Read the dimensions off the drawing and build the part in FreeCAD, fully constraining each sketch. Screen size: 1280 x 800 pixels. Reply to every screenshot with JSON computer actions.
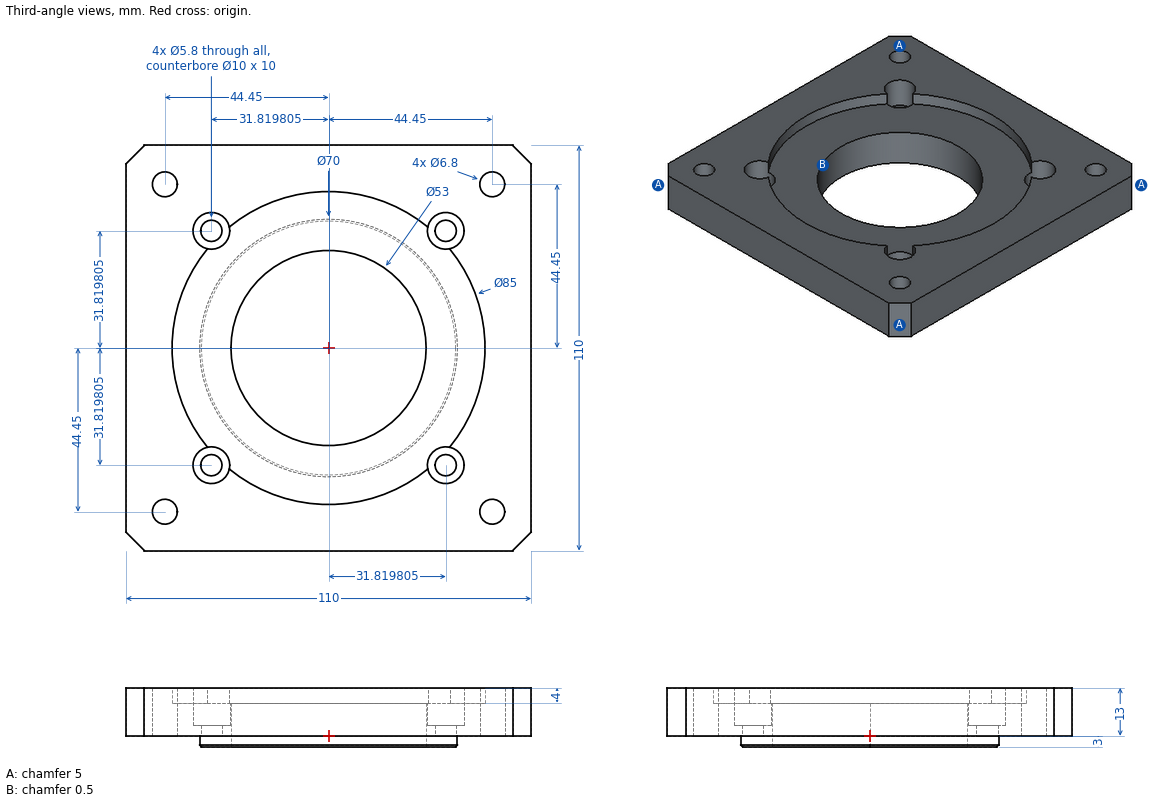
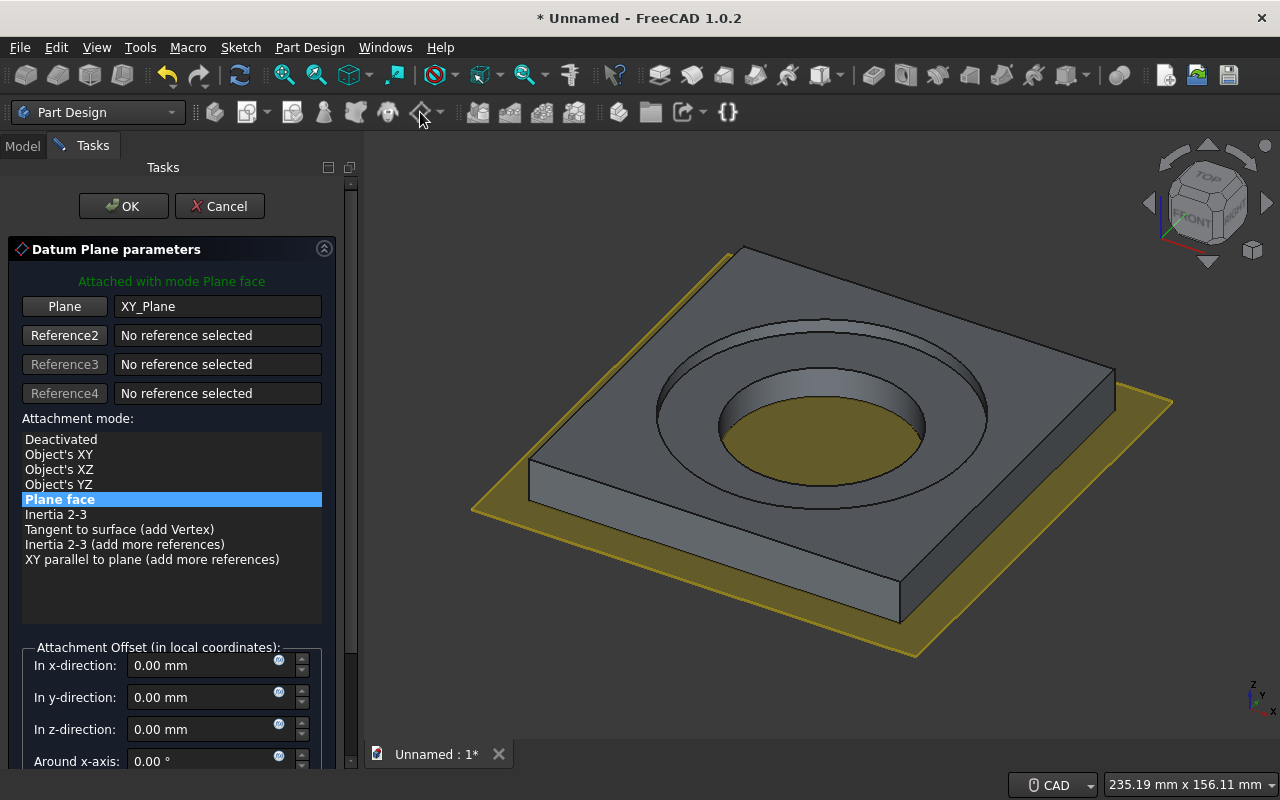
{"action": "triple_click", "coordinate": [210, 729]}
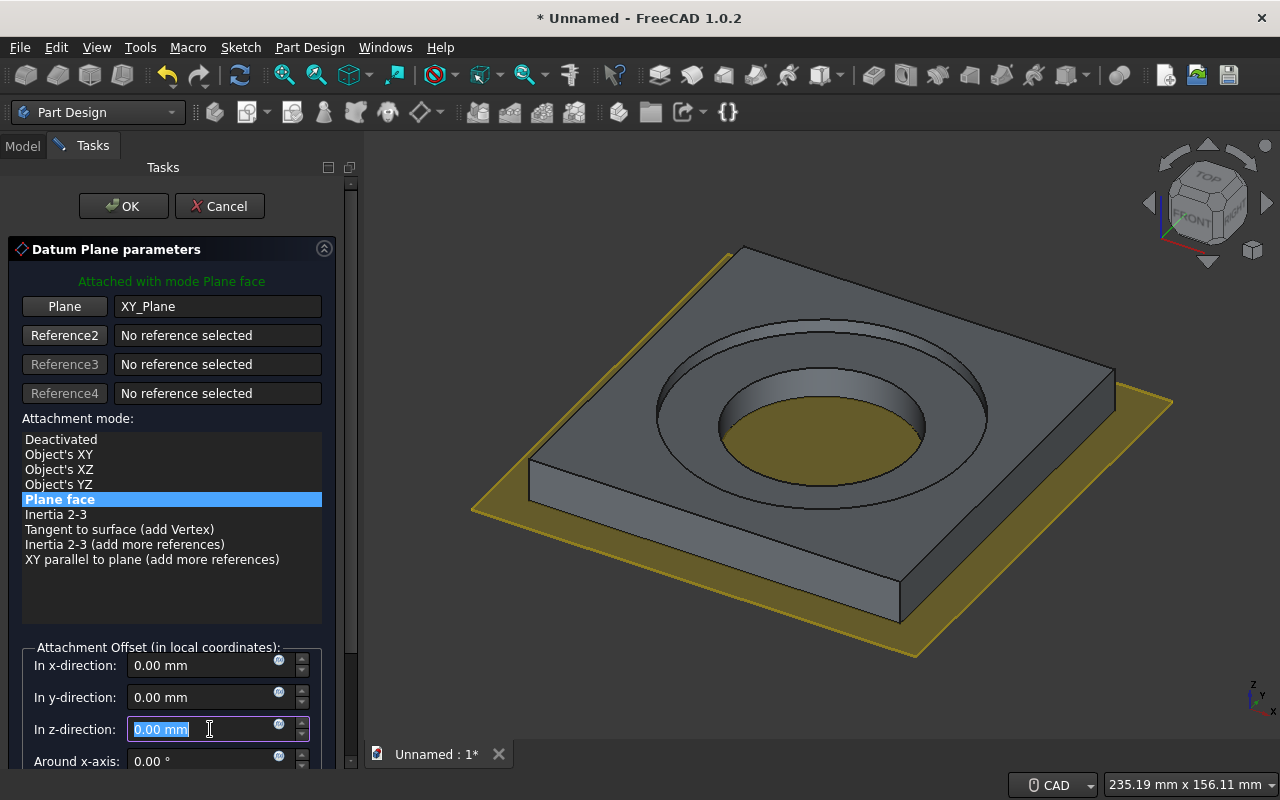
{"action": "type", "text": "-3"}
{"action": "key", "text": "Tab"}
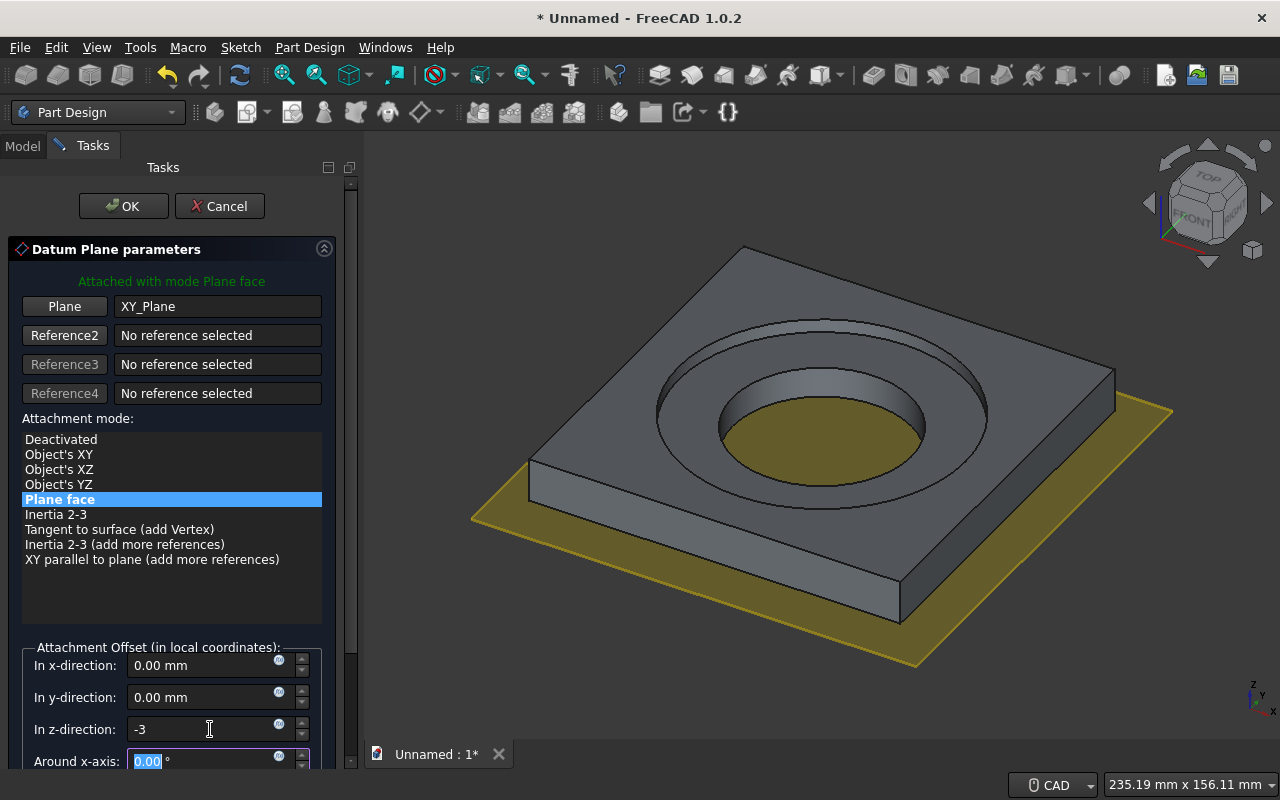
{"action": "left_click", "coordinate": [124, 206]}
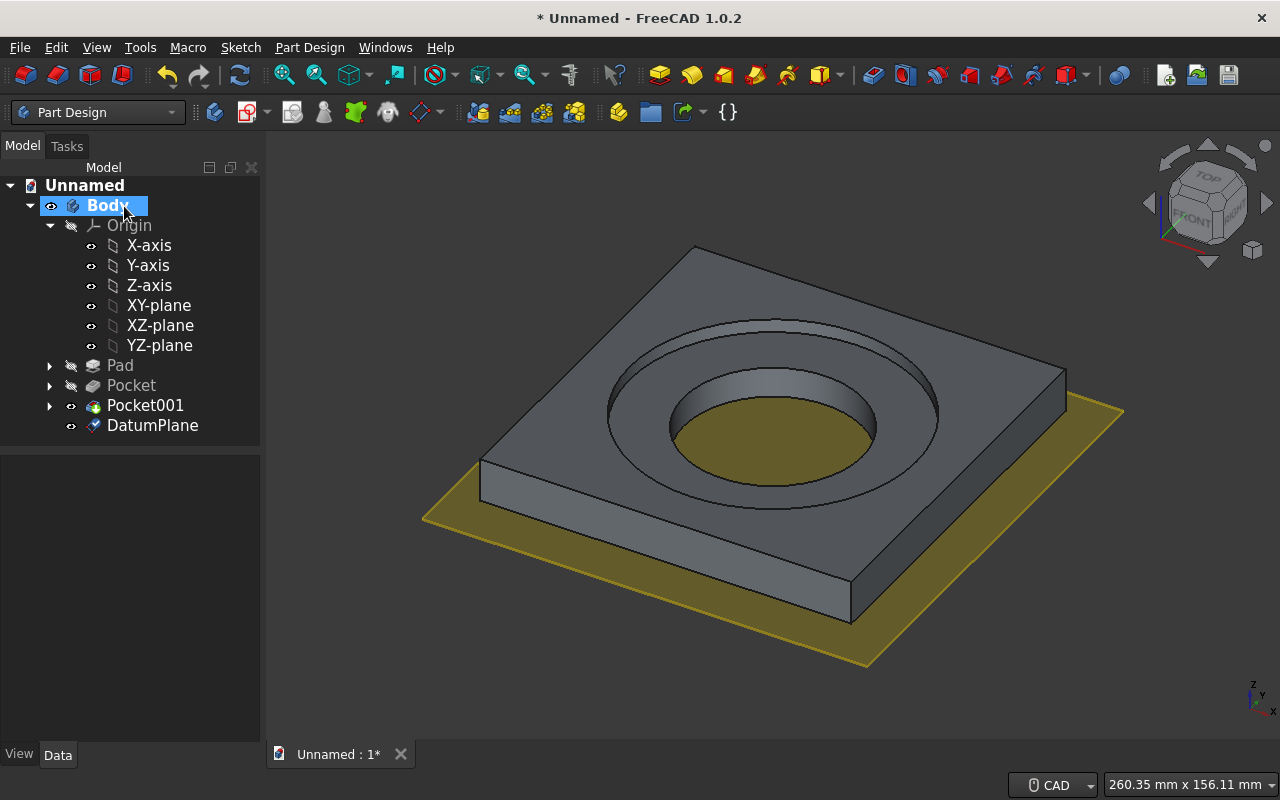
{"action": "left_click", "coordinate": [116, 426]}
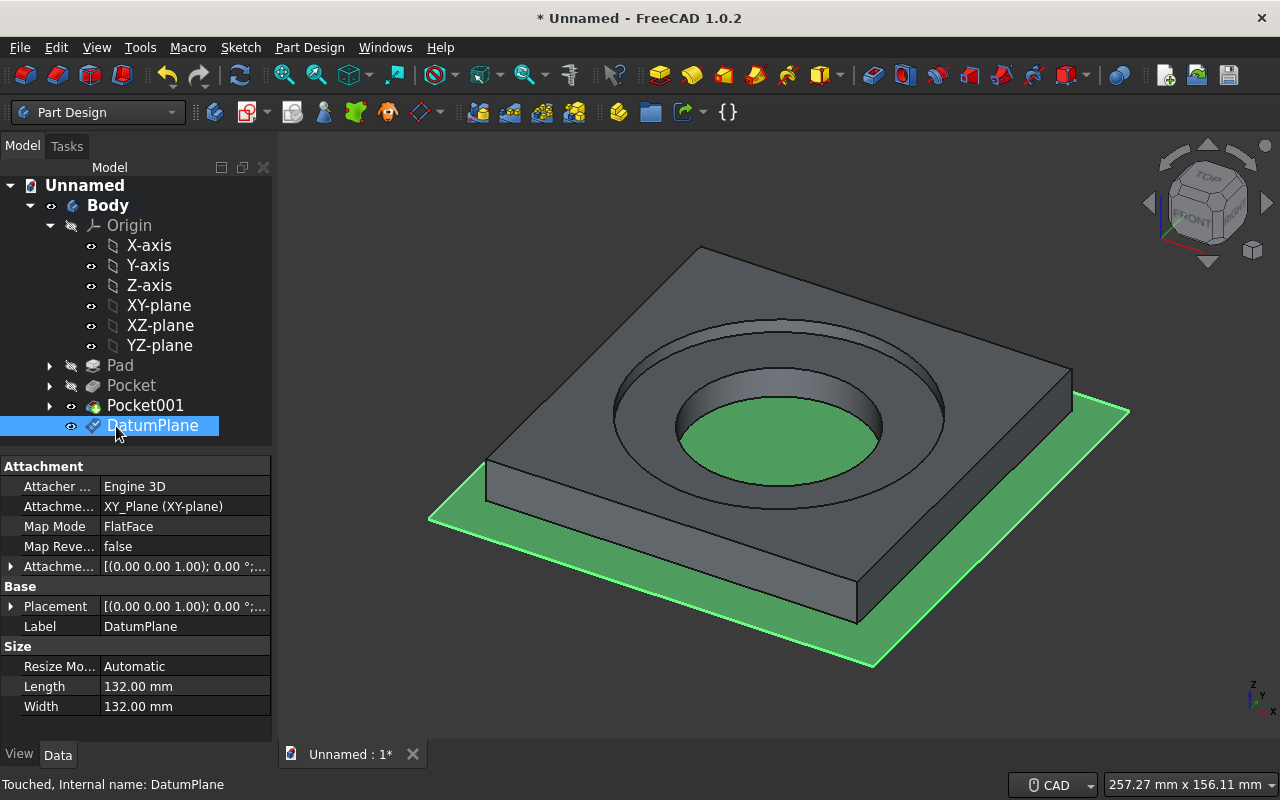
{"action": "left_click", "coordinate": [248, 112]}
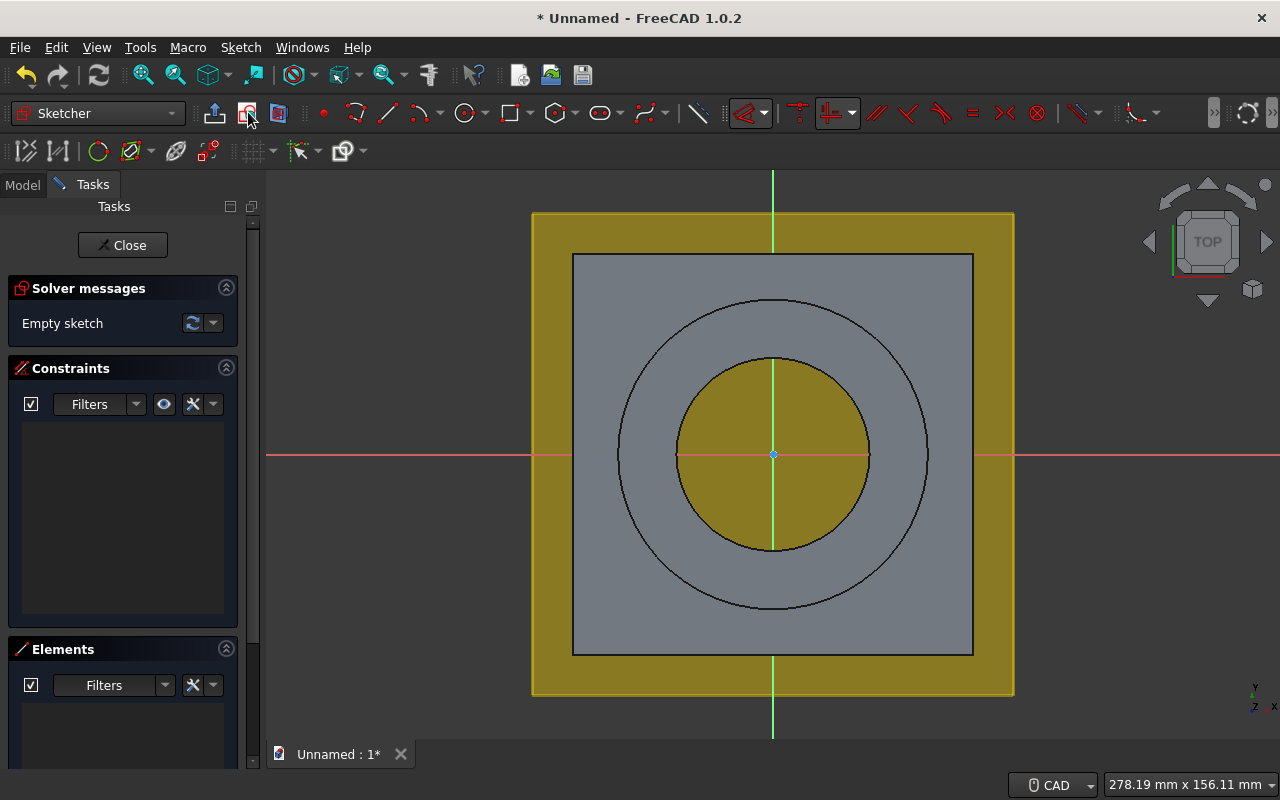
{"action": "left_click", "coordinate": [280, 114]}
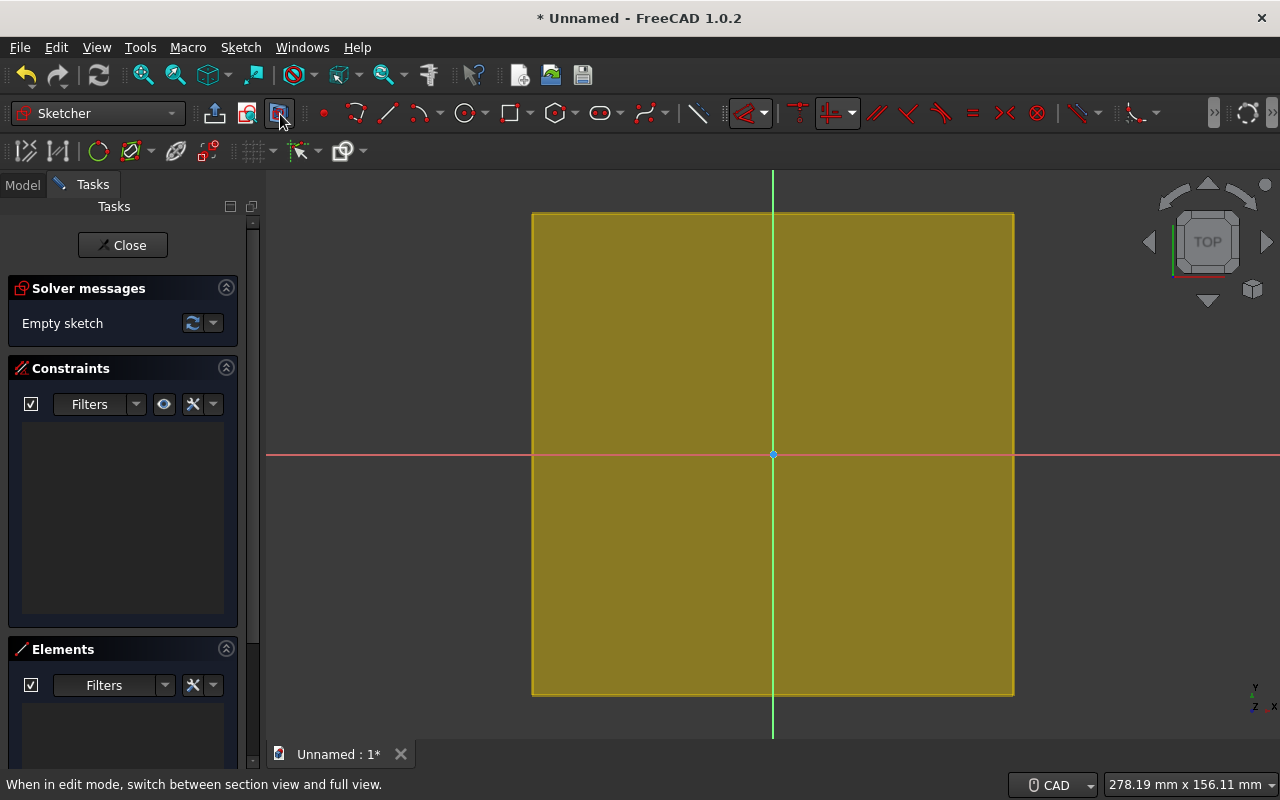
{"action": "scroll", "coordinate": [912, 455], "scroll_direction": "up", "scroll_amount": 2}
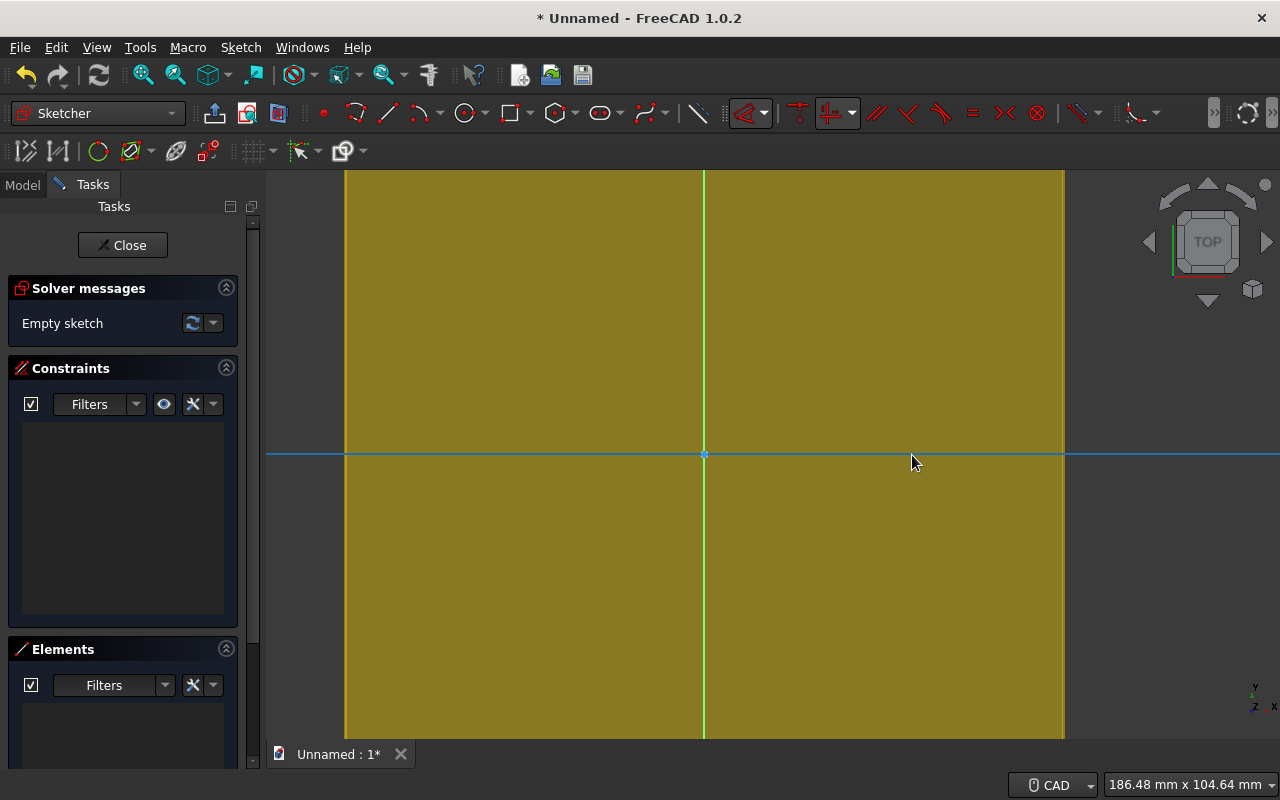
{"action": "key", "text": "g c"}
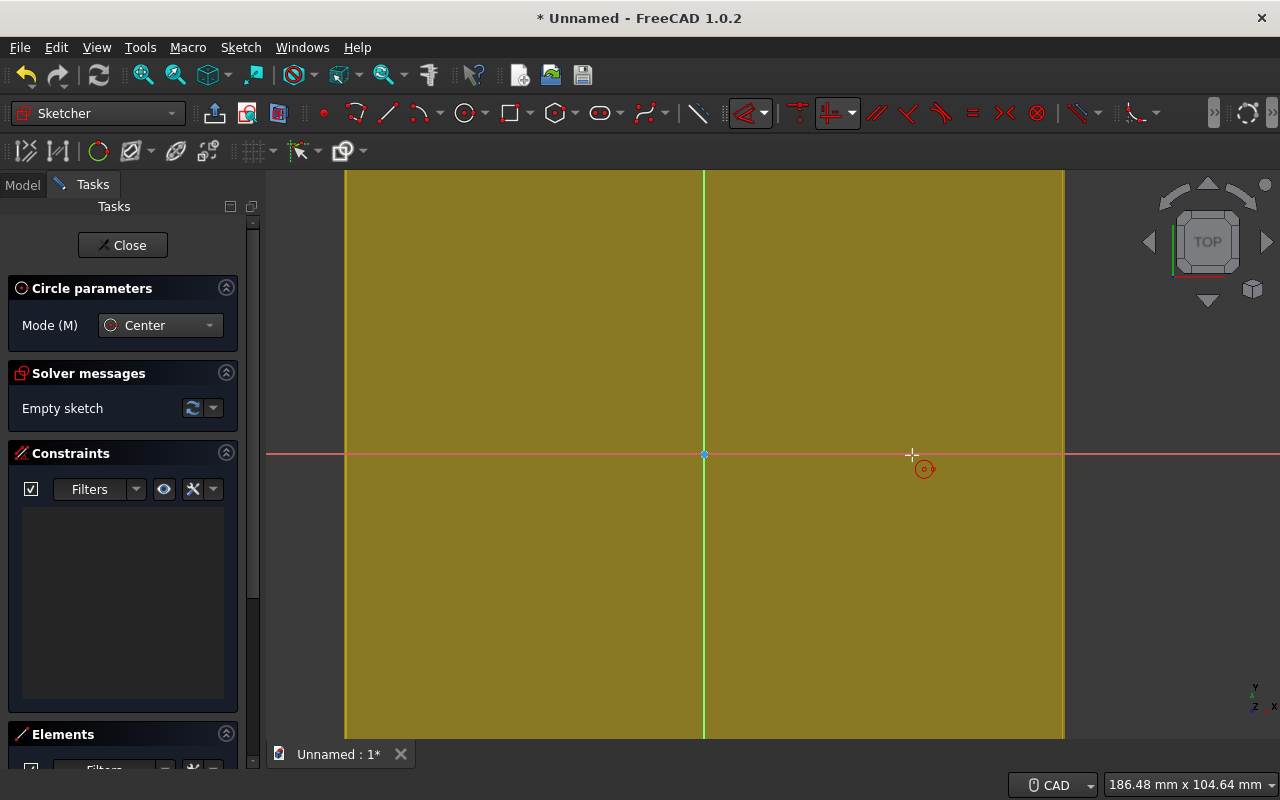
{"action": "left_click", "coordinate": [704, 454]}
{"action": "left_click", "coordinate": [839, 319]}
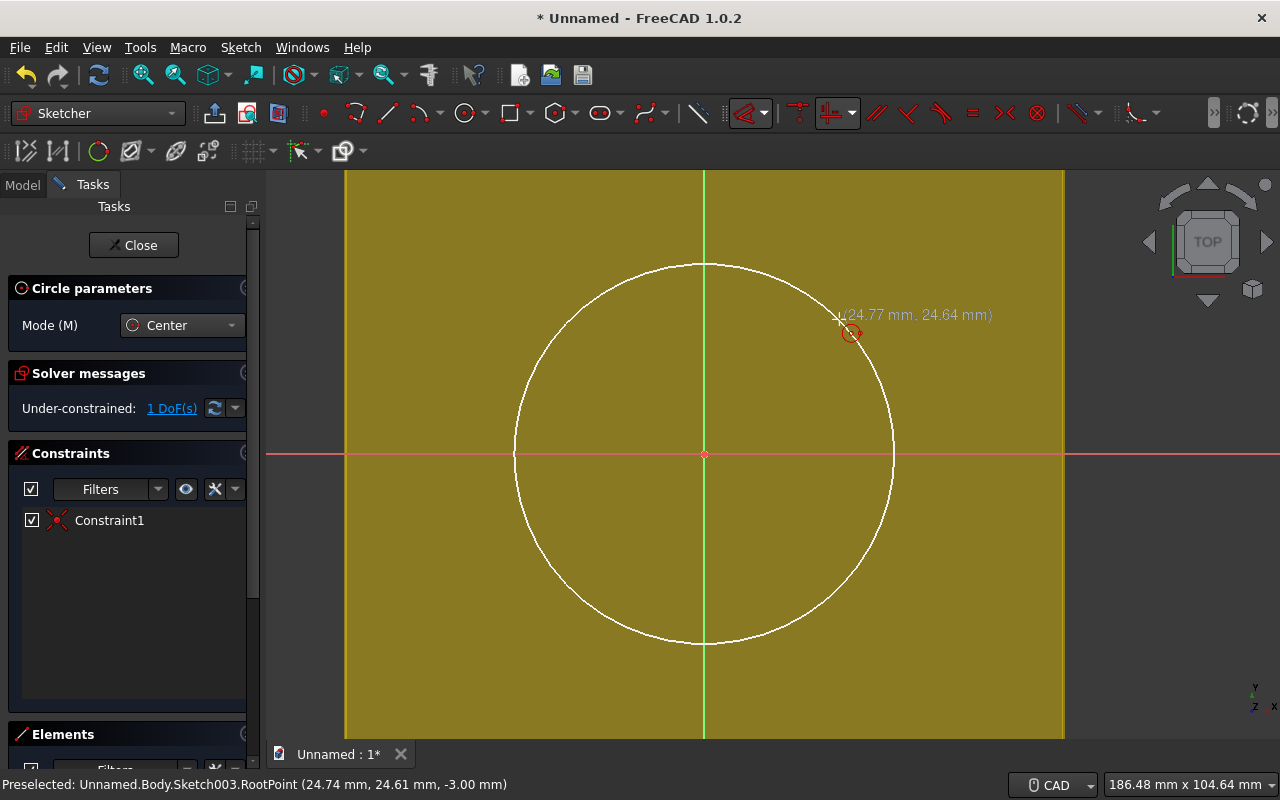
{"action": "left_click", "coordinate": [704, 454]}
{"action": "left_click", "coordinate": [806, 352]}
{"action": "key", "text": "Escape"}